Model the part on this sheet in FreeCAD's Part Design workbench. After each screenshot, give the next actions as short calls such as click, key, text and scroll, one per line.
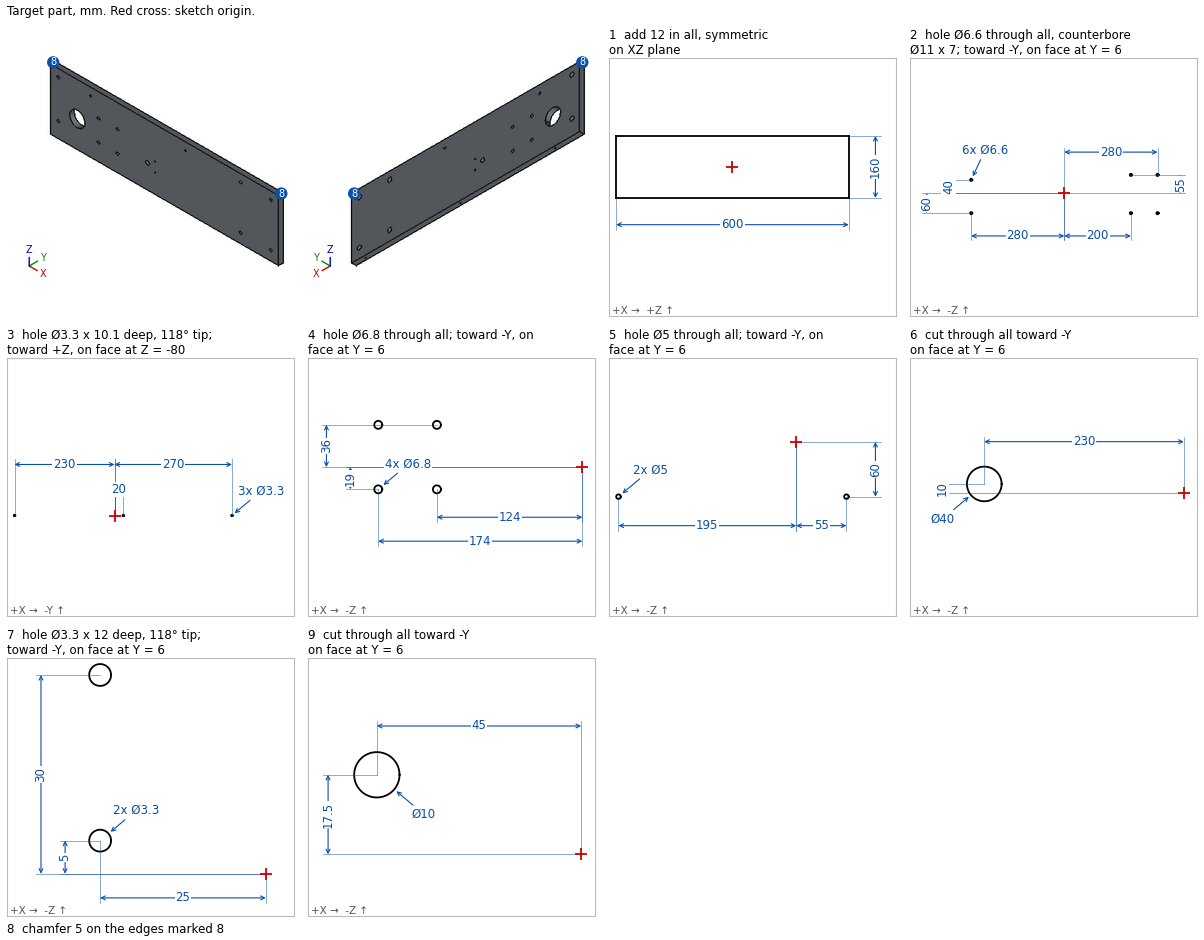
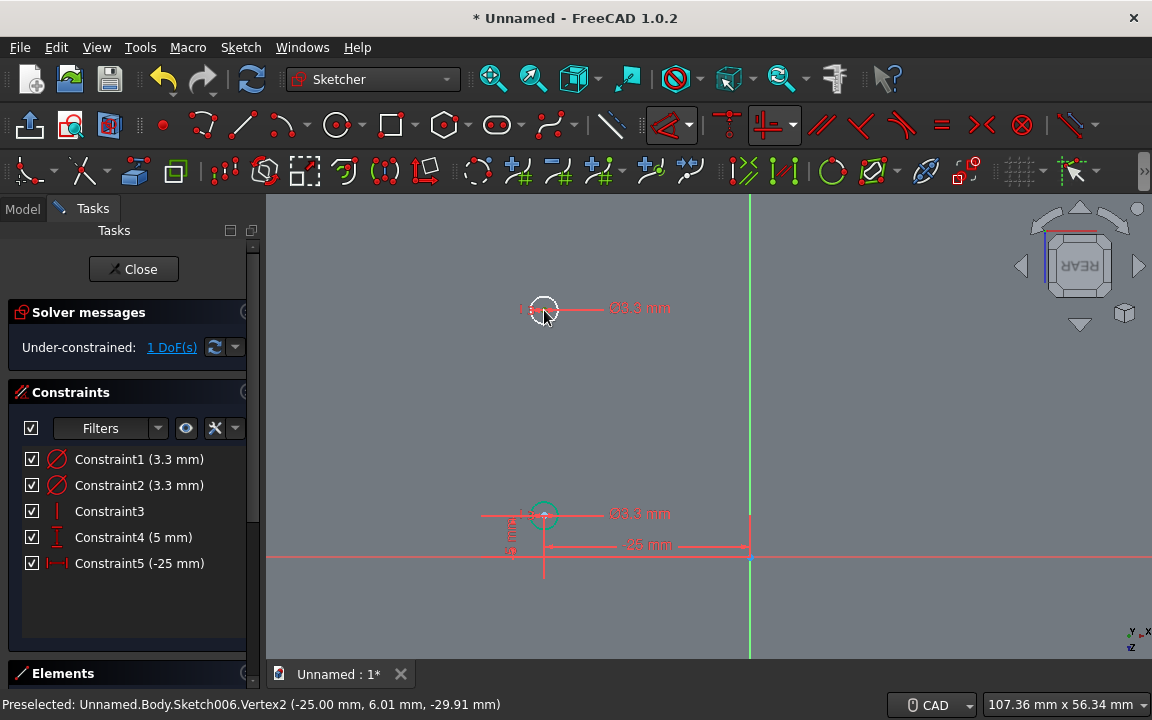
click(692, 126)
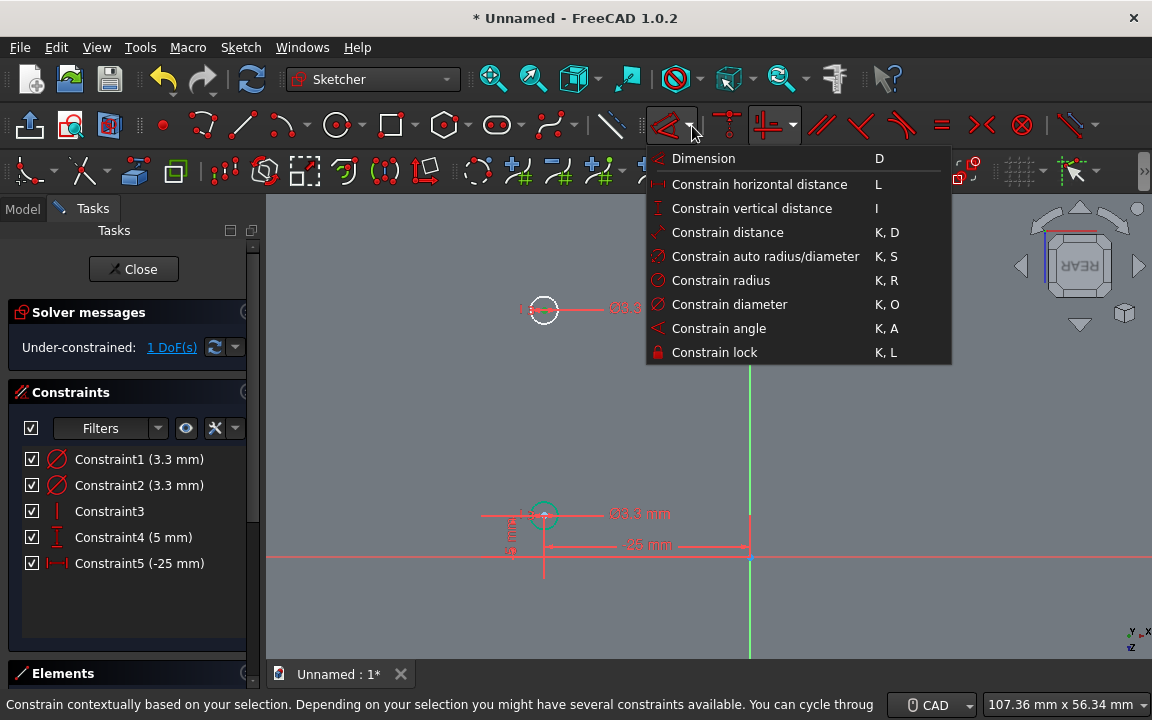
click(799, 208)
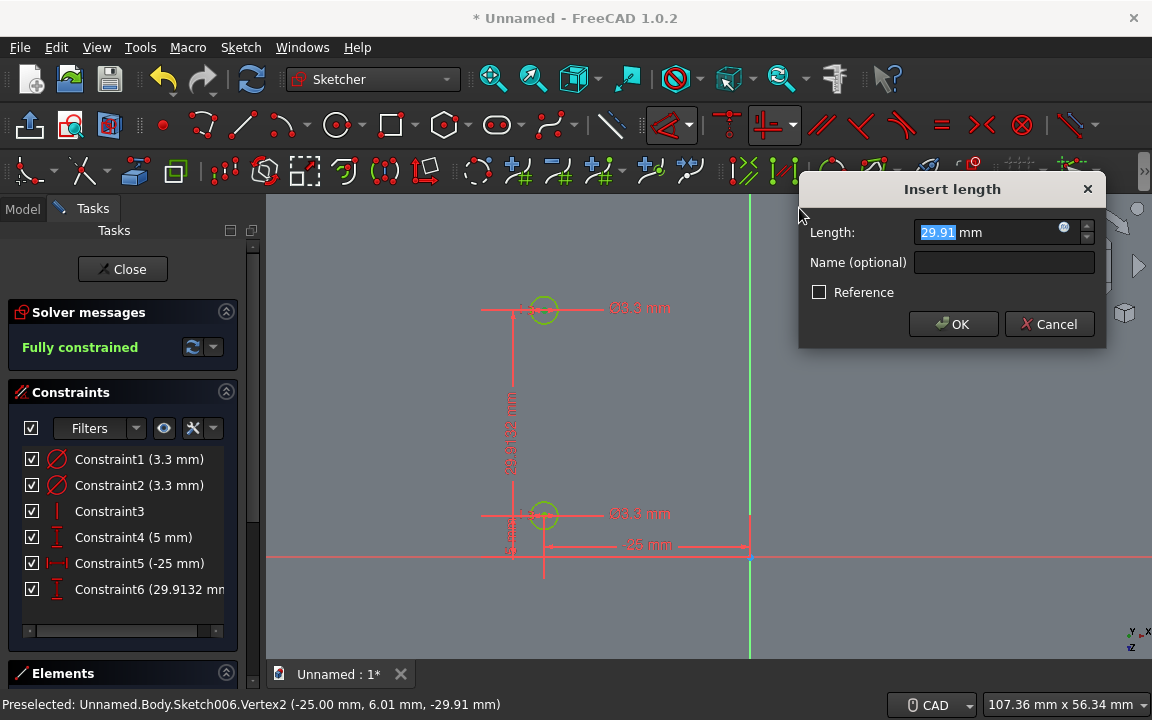
text(30)
key(Return)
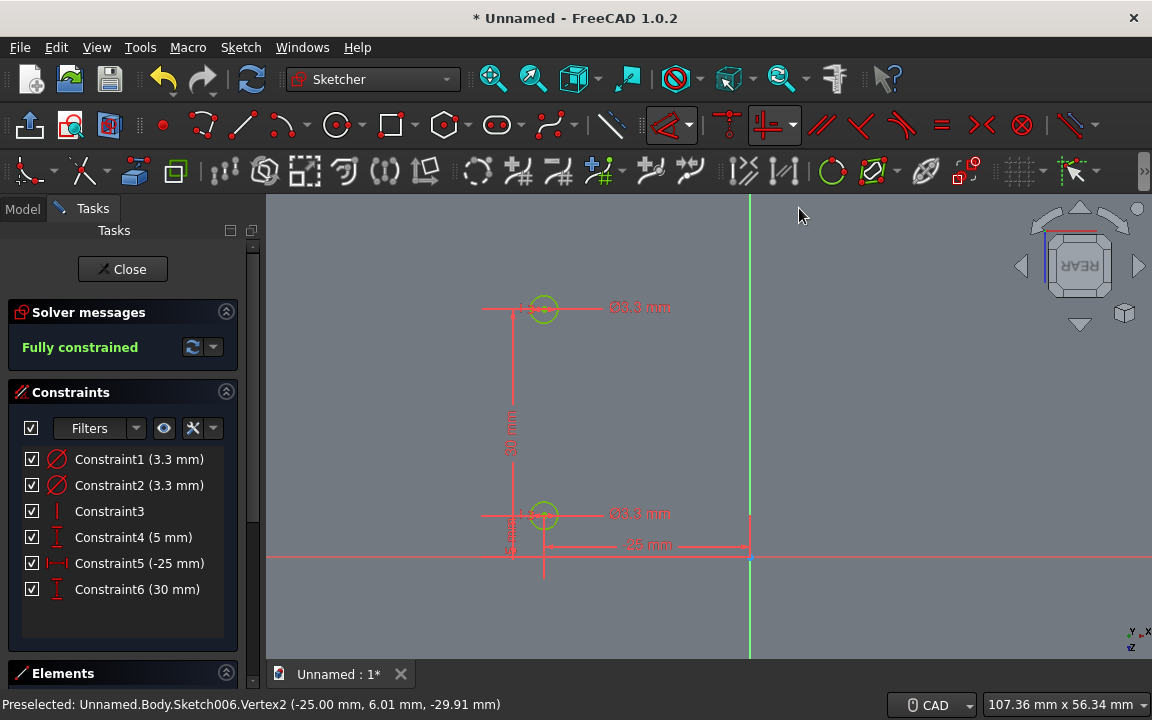
click(123, 269)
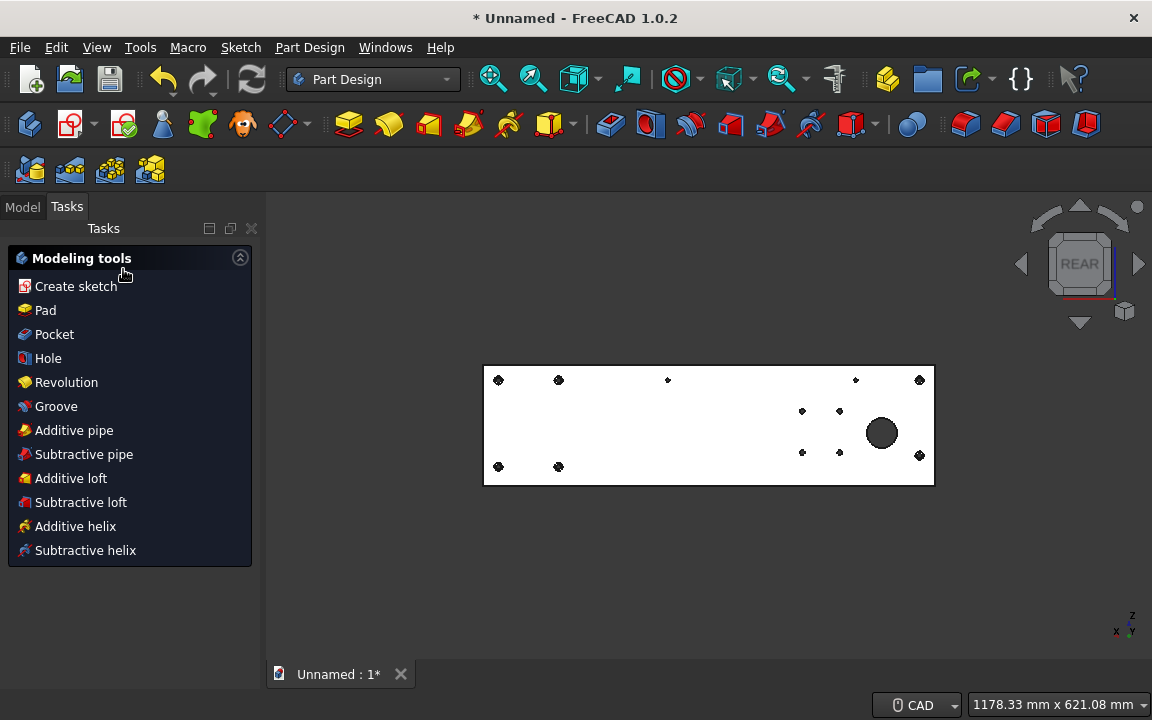
click(652, 124)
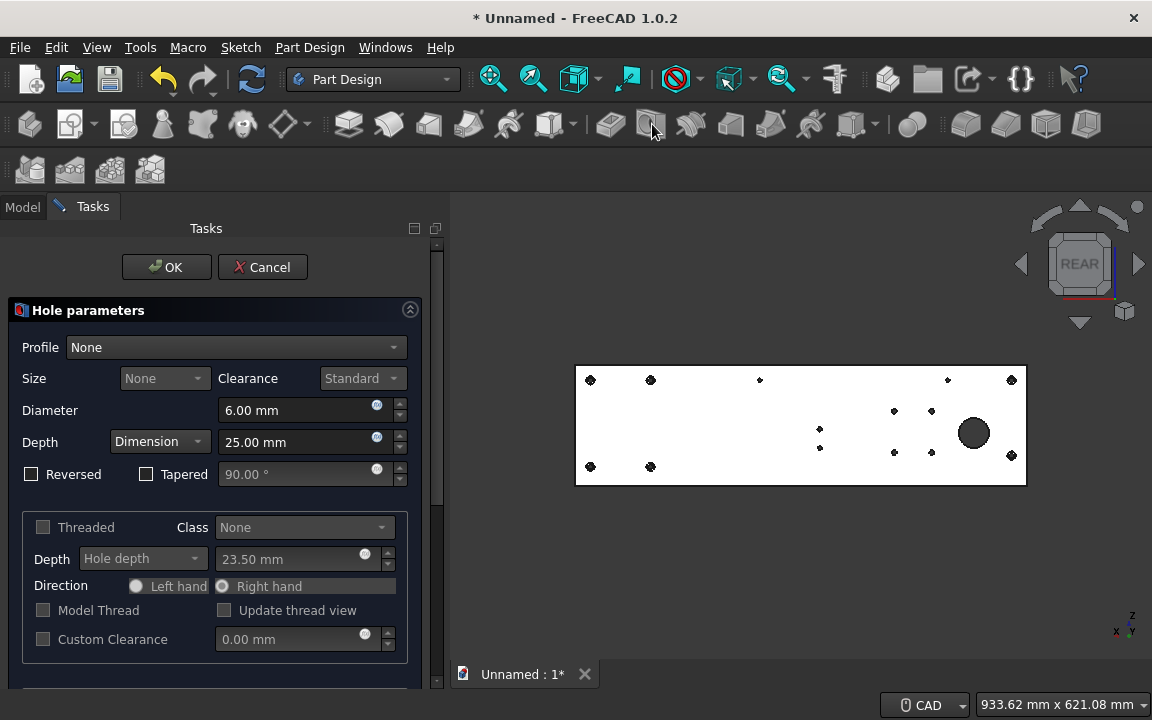
triple_click(305, 410)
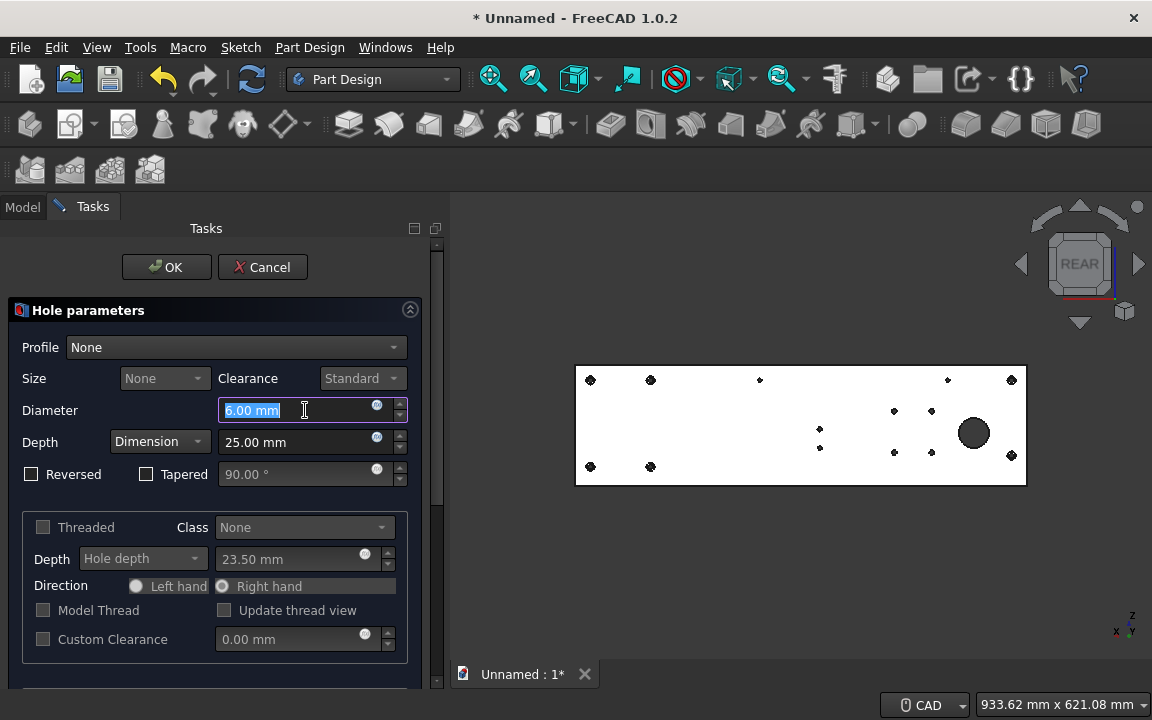
text(3.3)
key(Tab)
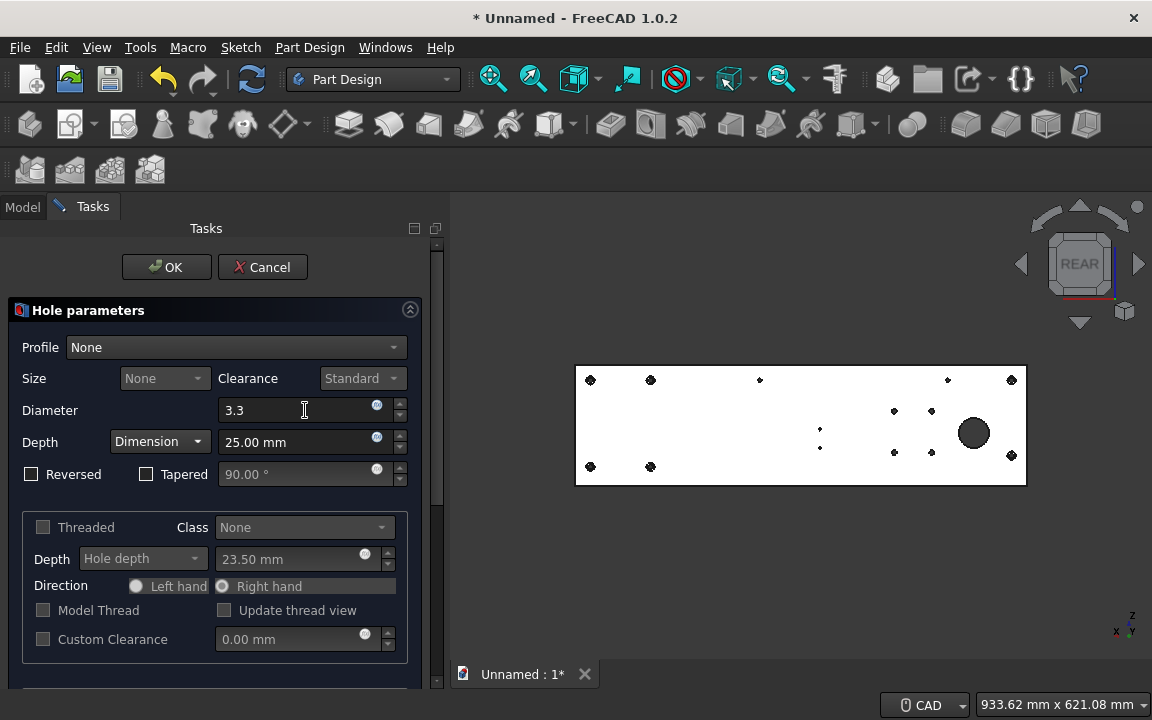
triple_click(305, 442)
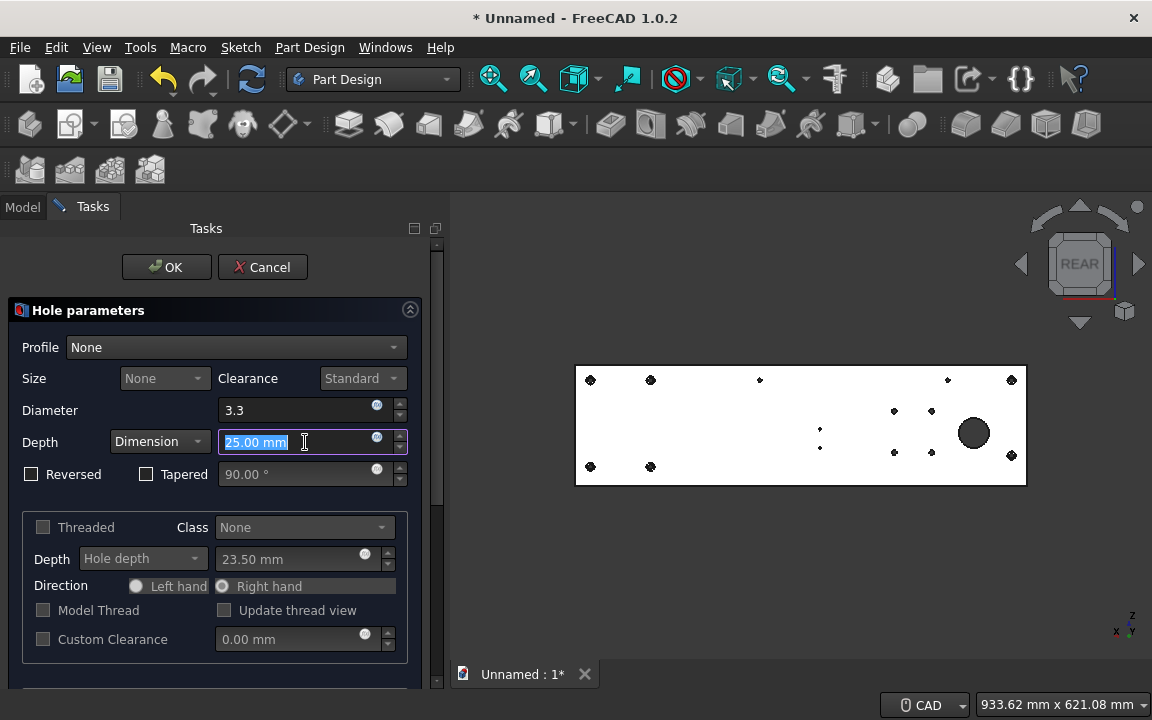
text(12)
key(Tab)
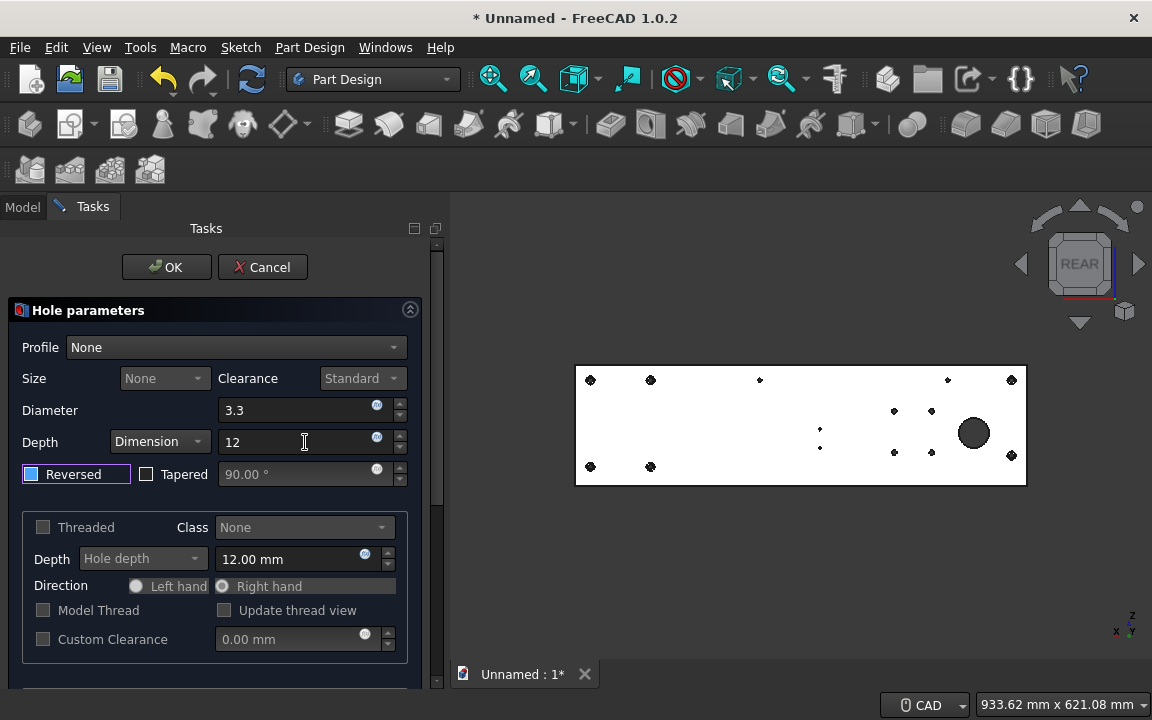
click(167, 267)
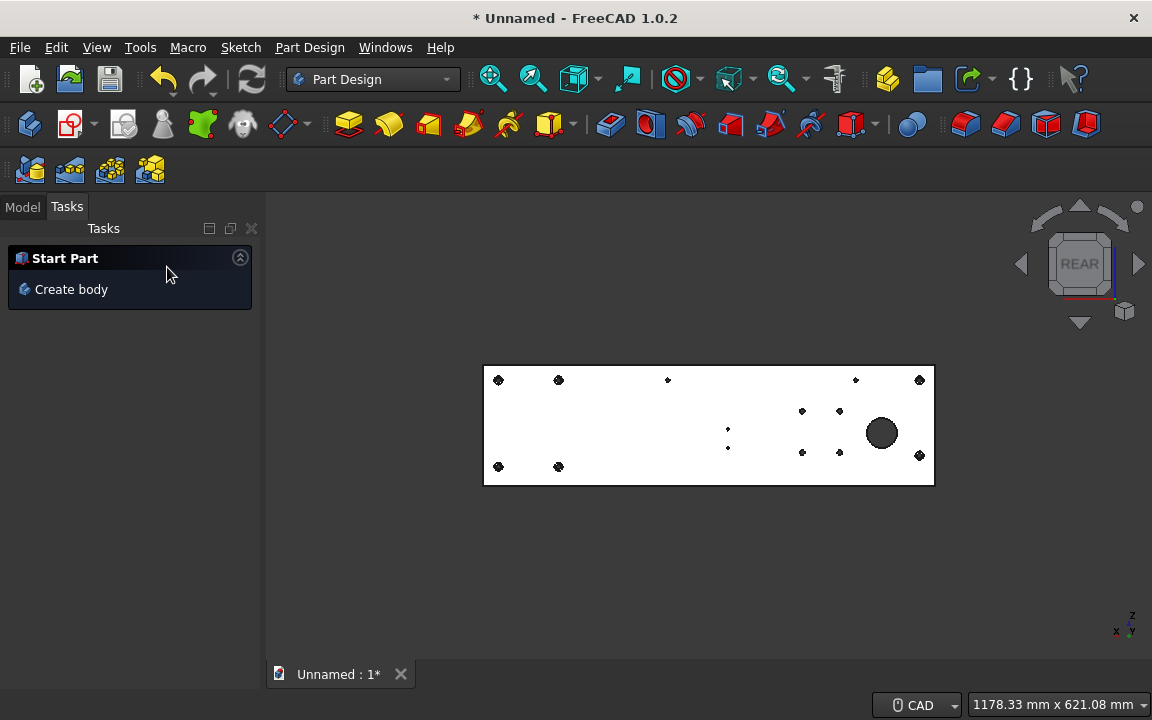
scroll(483, 364, up, 8)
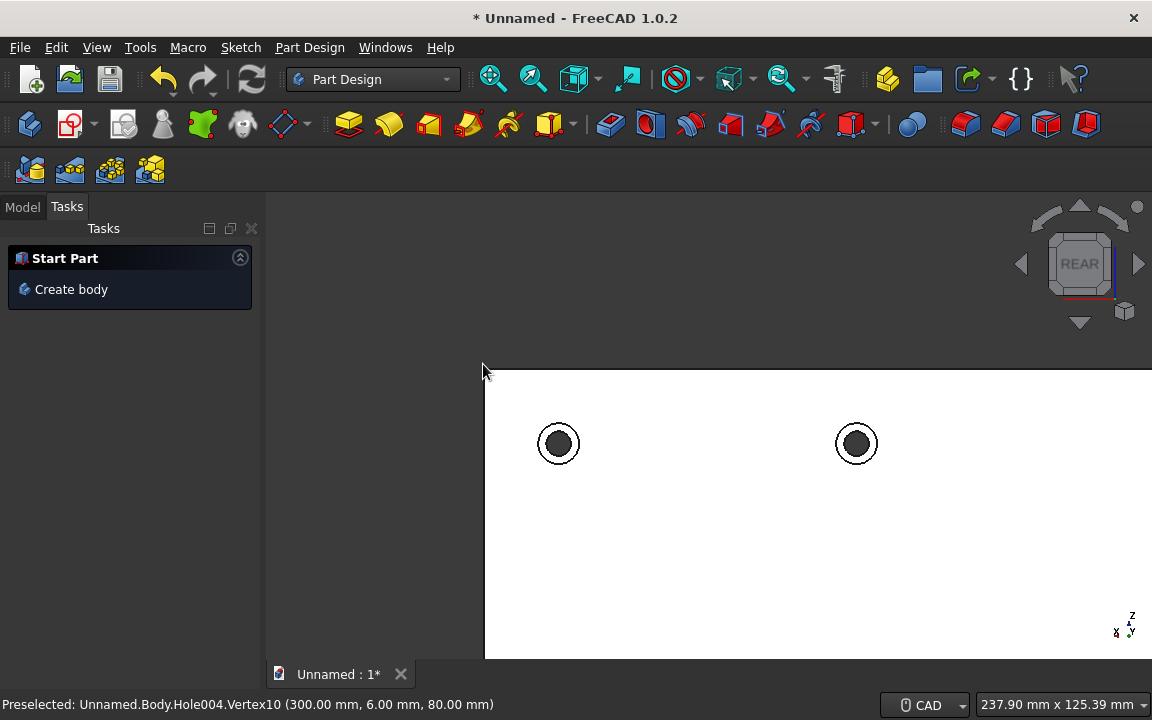
key(v)
key(f)